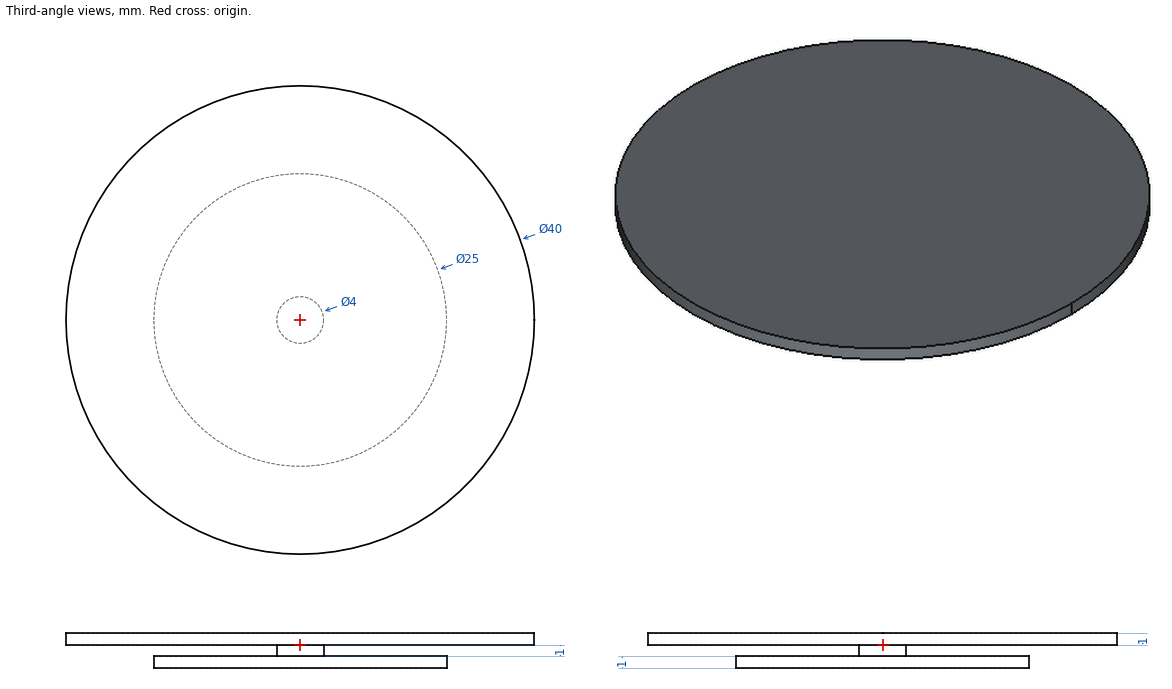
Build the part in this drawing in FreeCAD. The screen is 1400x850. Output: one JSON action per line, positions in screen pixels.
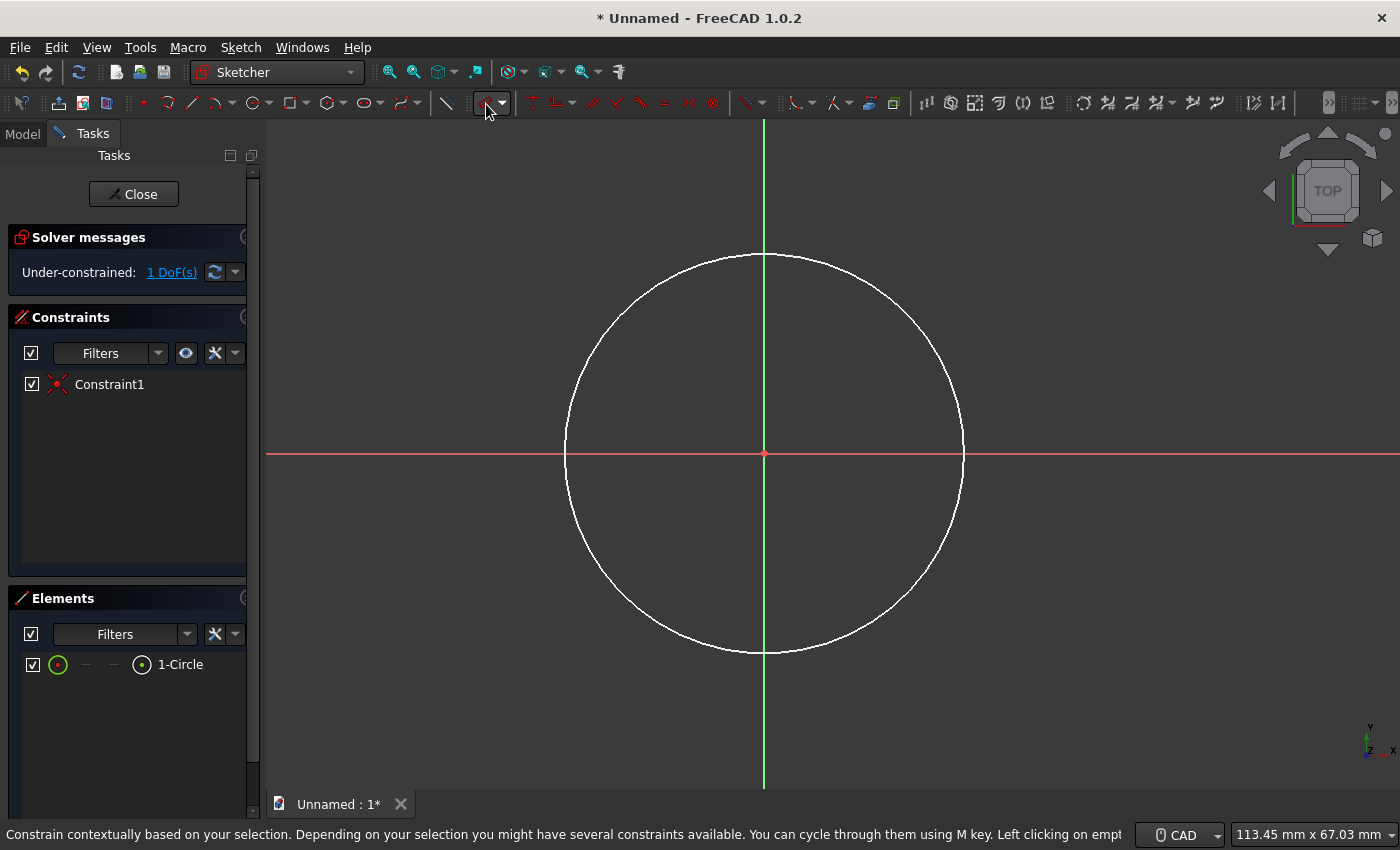
{"action": "left_click", "coordinate": [905, 312]}
{"action": "left_click", "coordinate": [928, 289]}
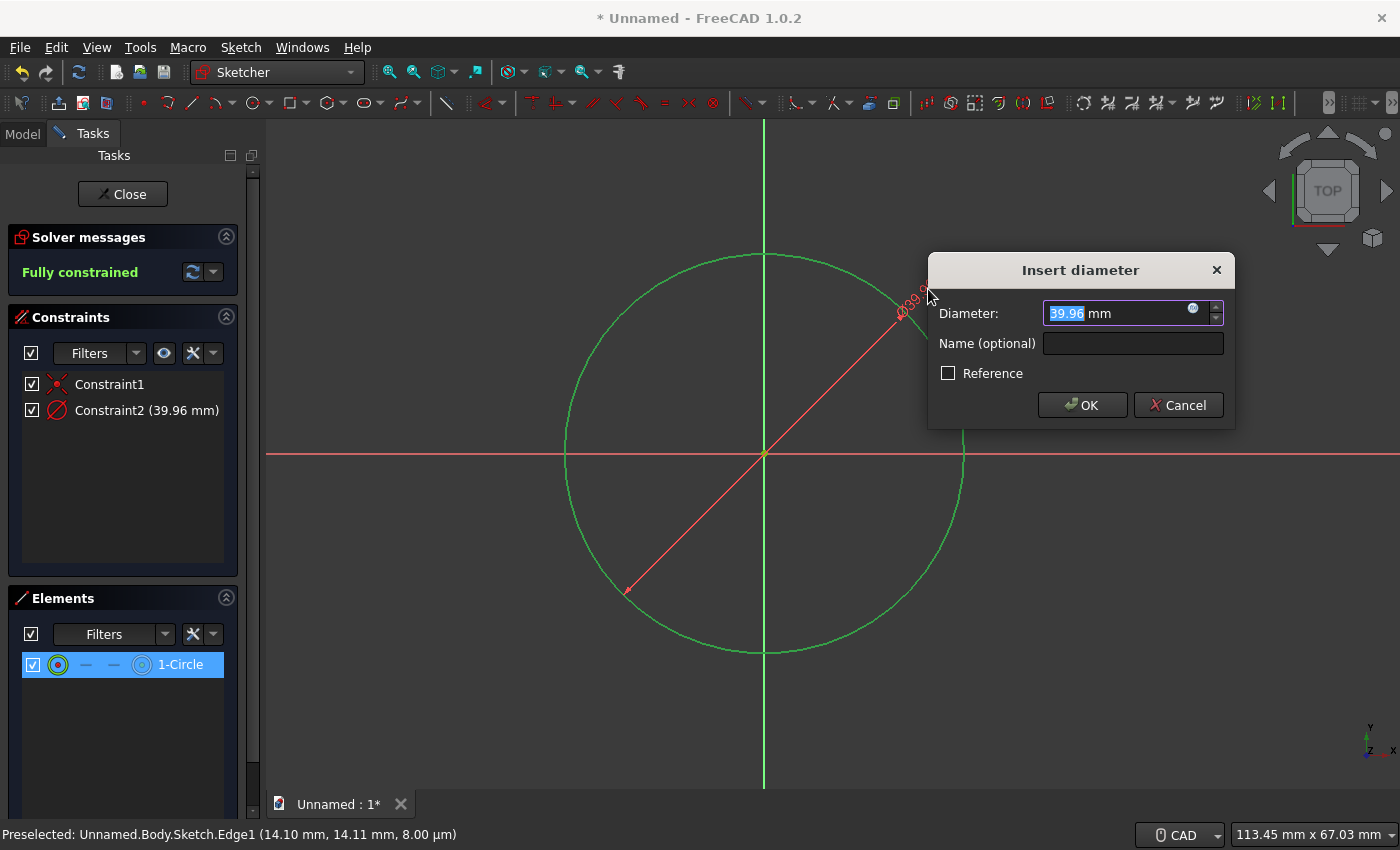
{"action": "type", "text": "40"}
{"action": "key", "text": "Return"}
{"action": "key", "text": "Escape"}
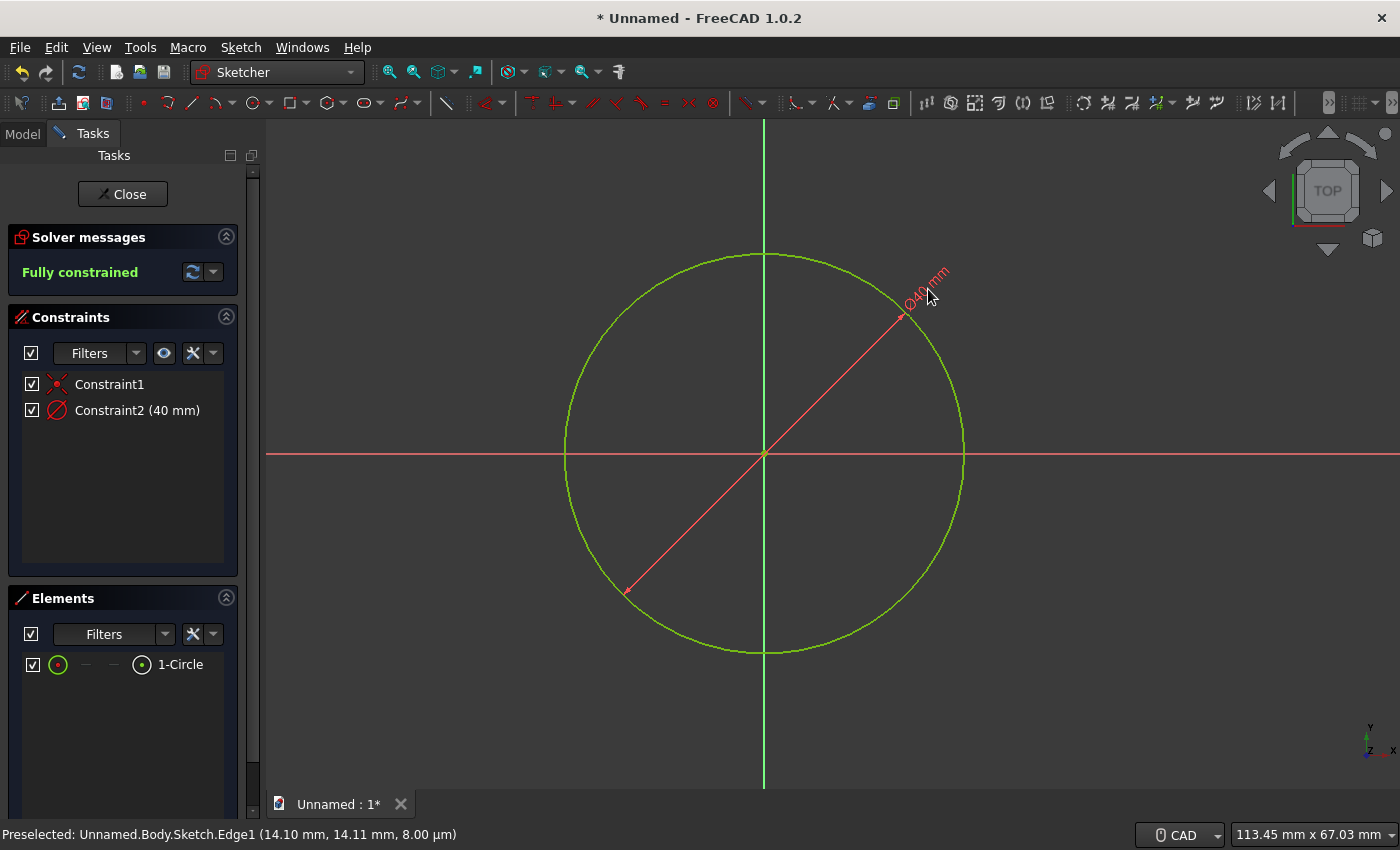
{"action": "left_click", "coordinate": [123, 194]}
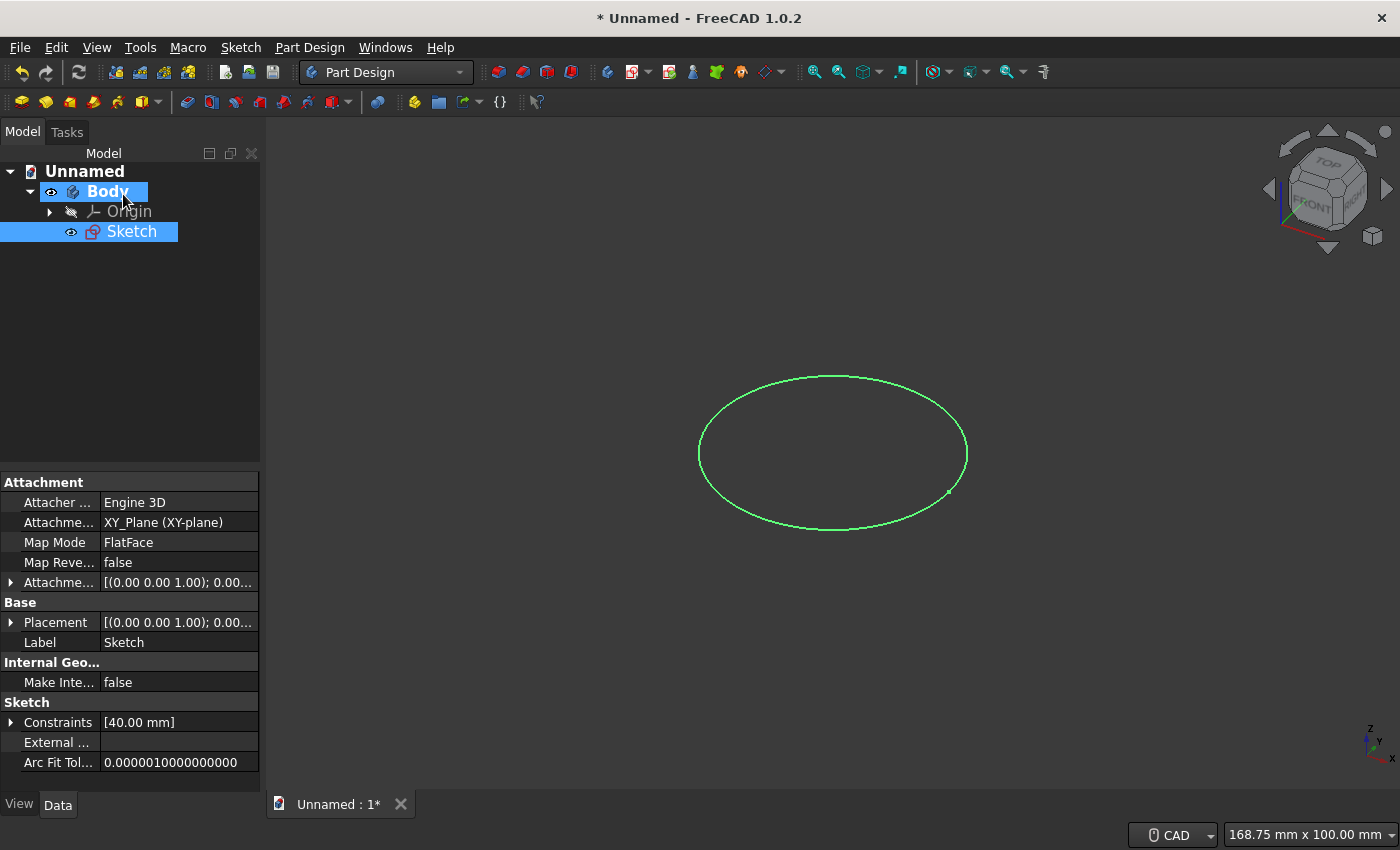
{"action": "left_click", "coordinate": [22, 102]}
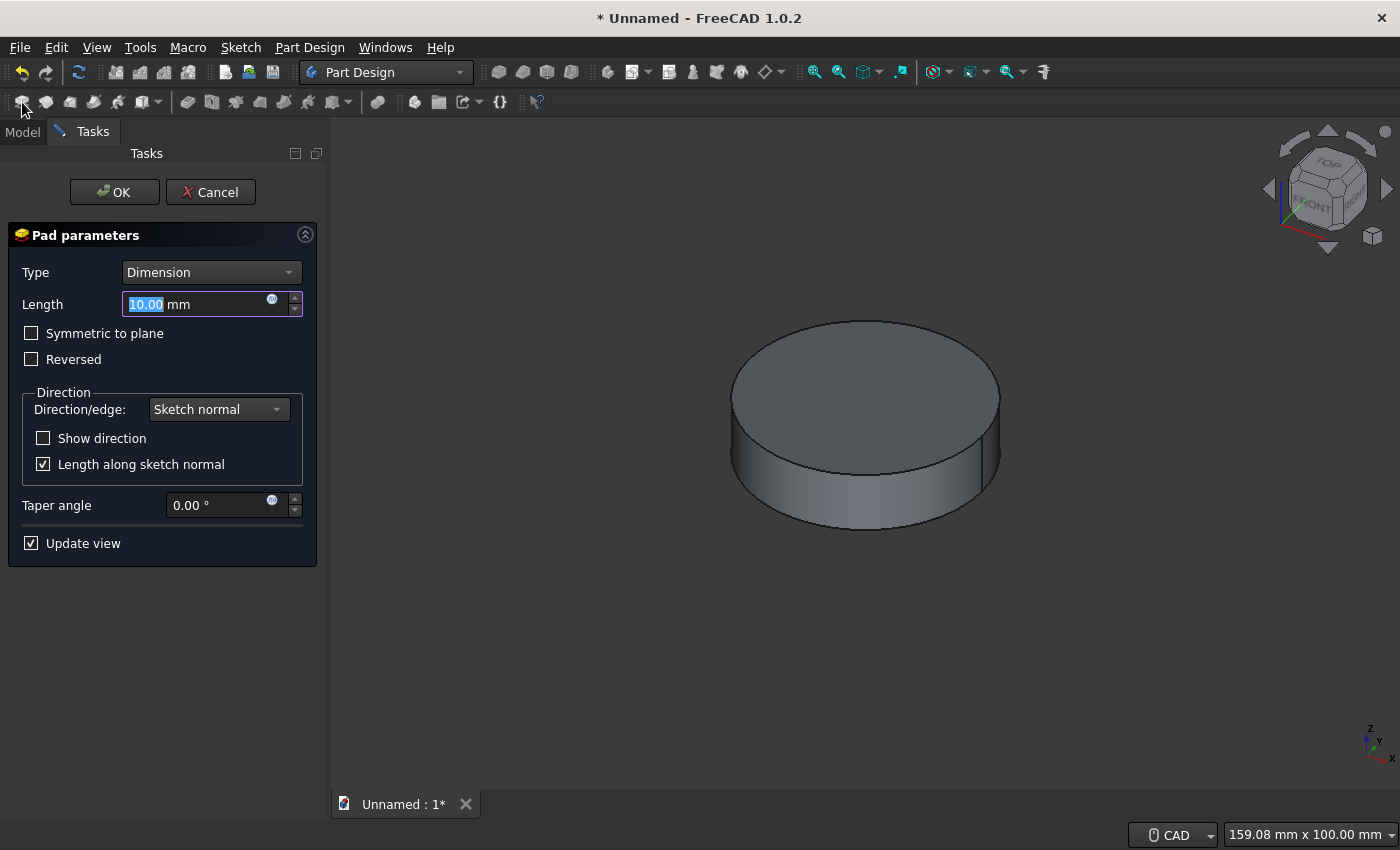
{"action": "type", "text": "1"}
{"action": "key", "text": "Tab"}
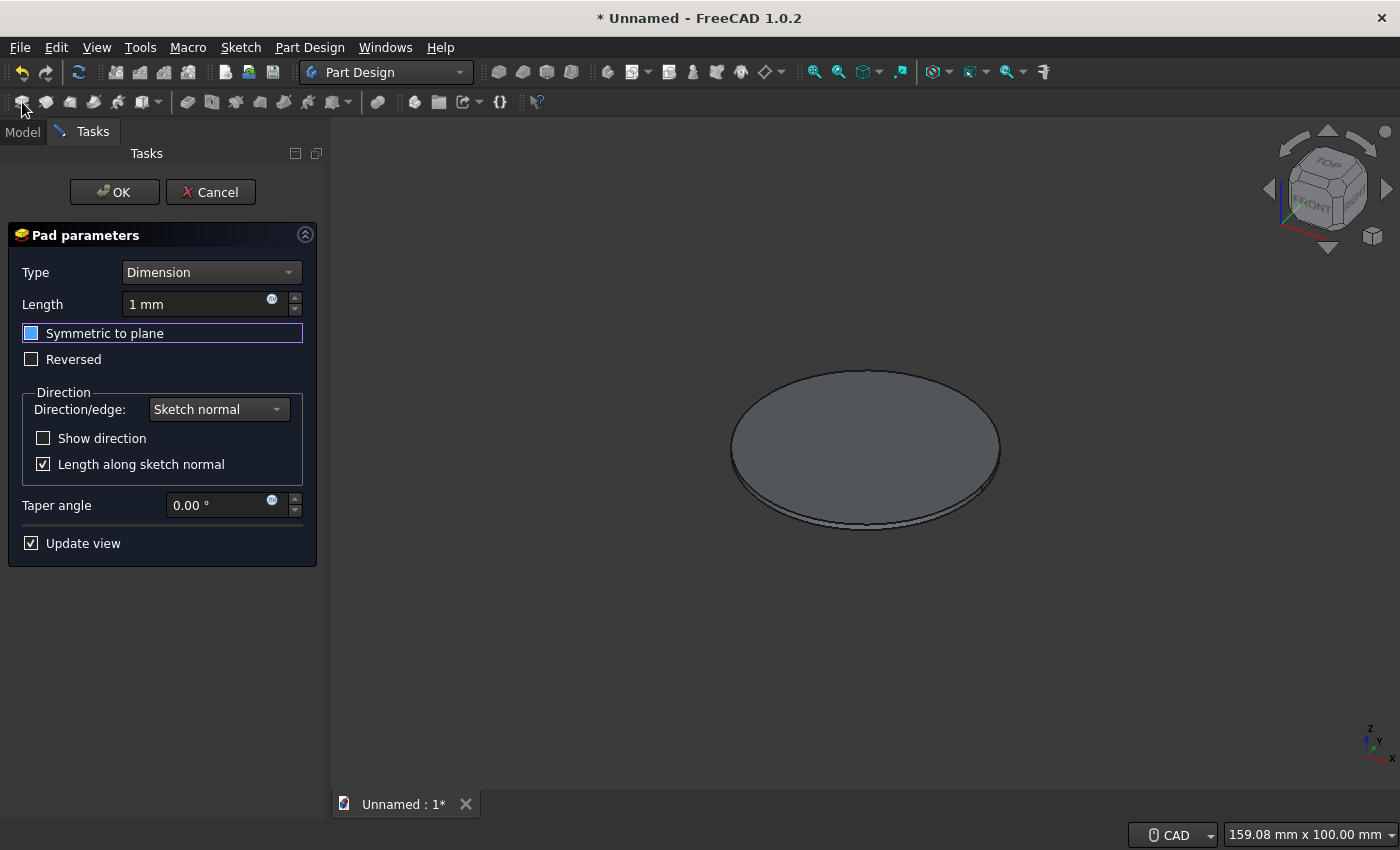
{"action": "left_click", "coordinate": [115, 192]}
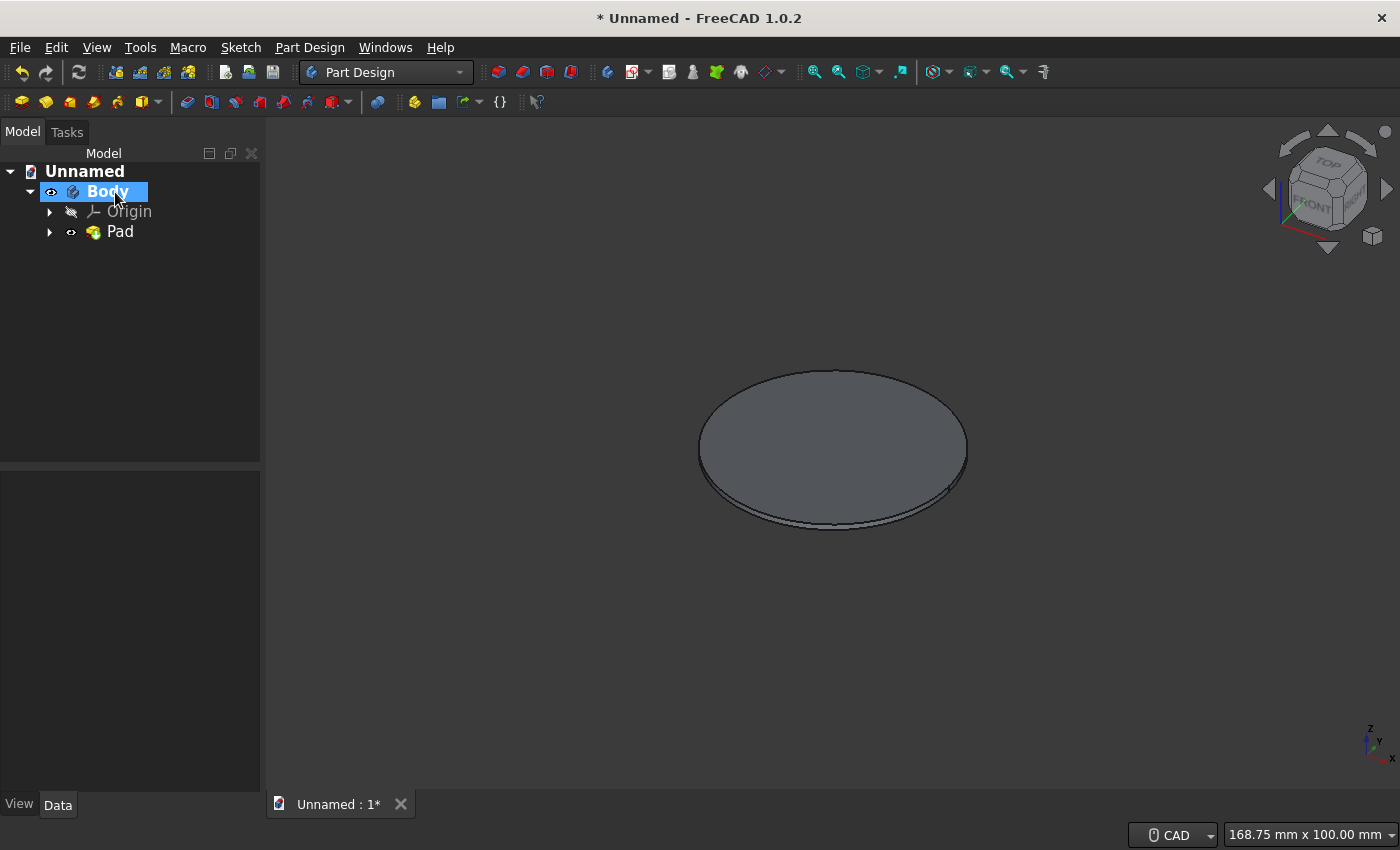
{"action": "left_click", "coordinate": [816, 72]}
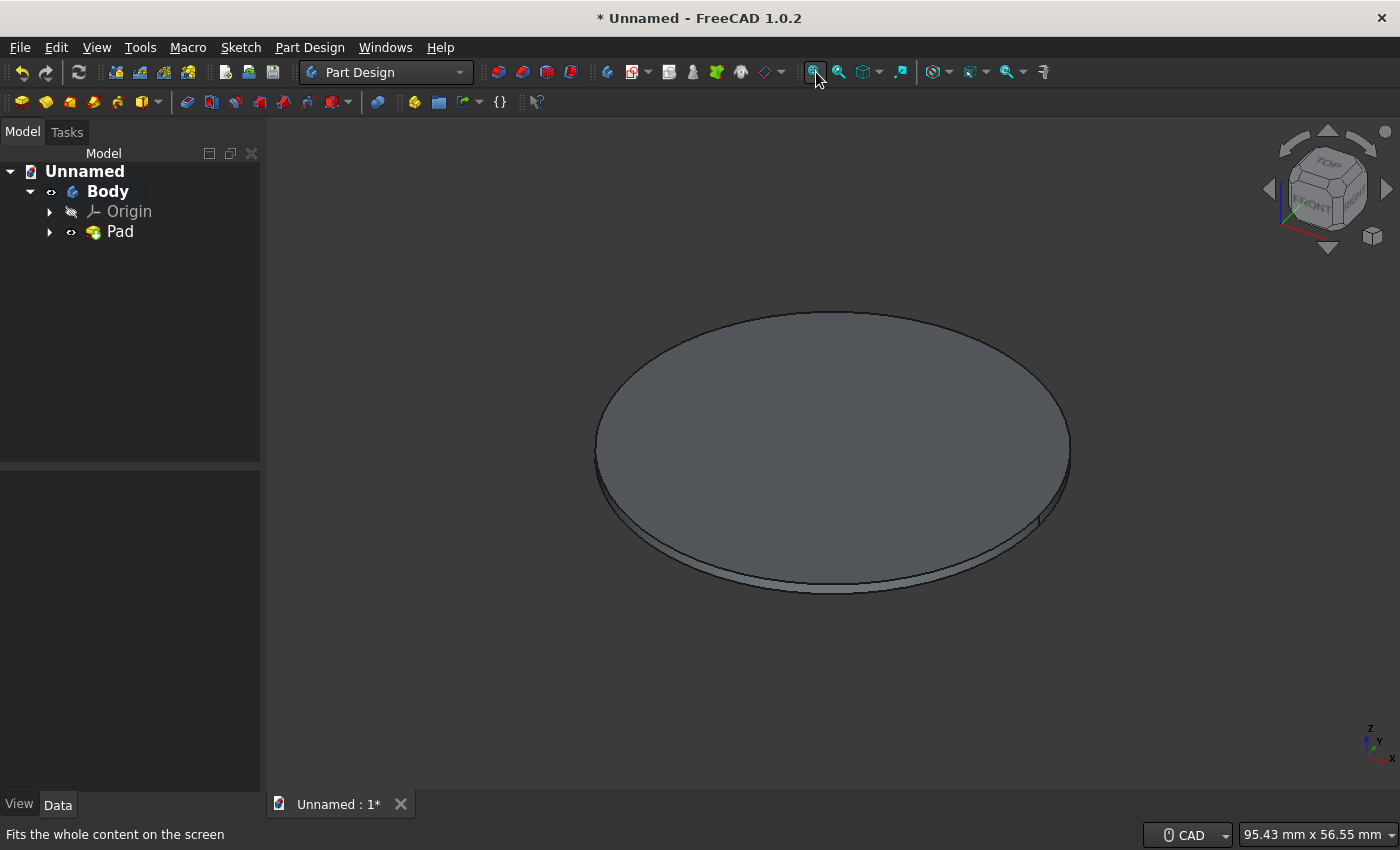
{"action": "key", "text": "5"}